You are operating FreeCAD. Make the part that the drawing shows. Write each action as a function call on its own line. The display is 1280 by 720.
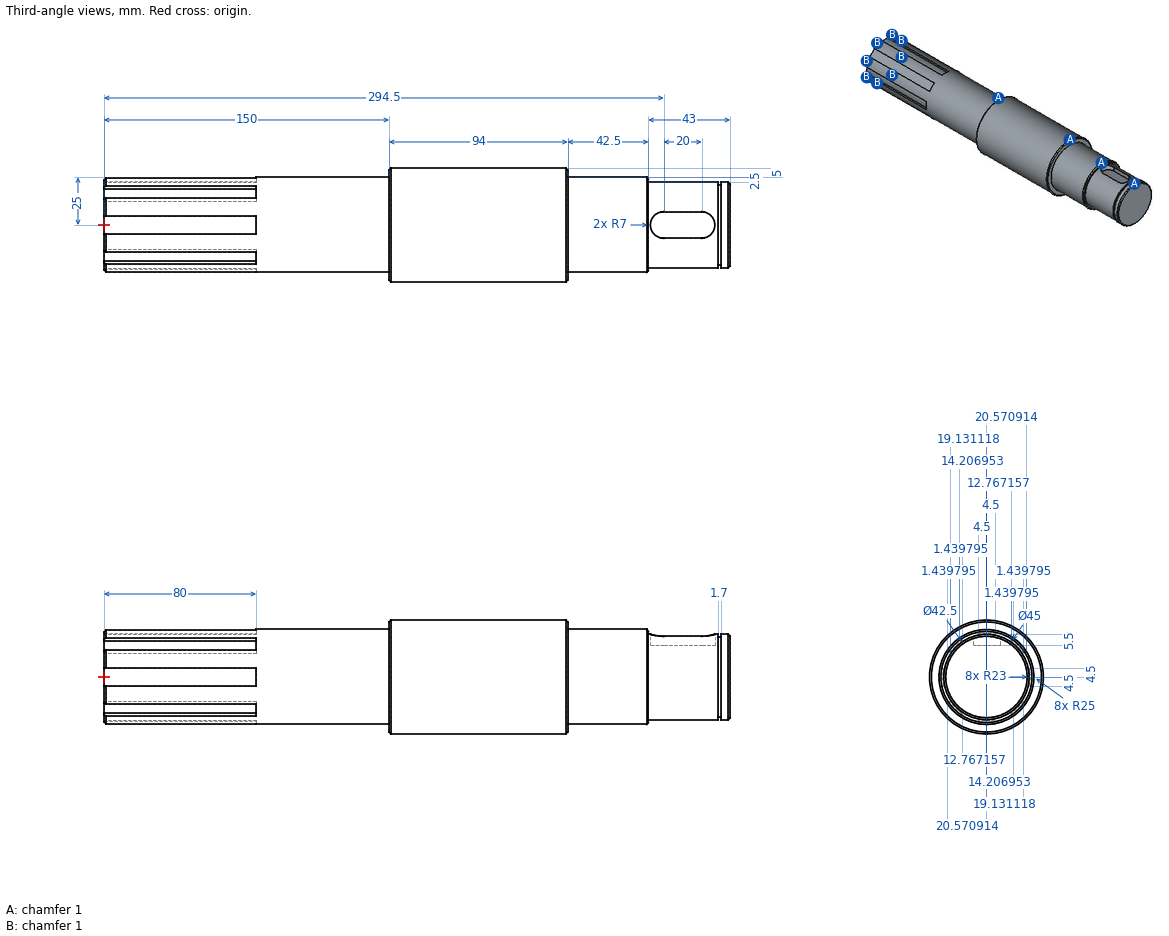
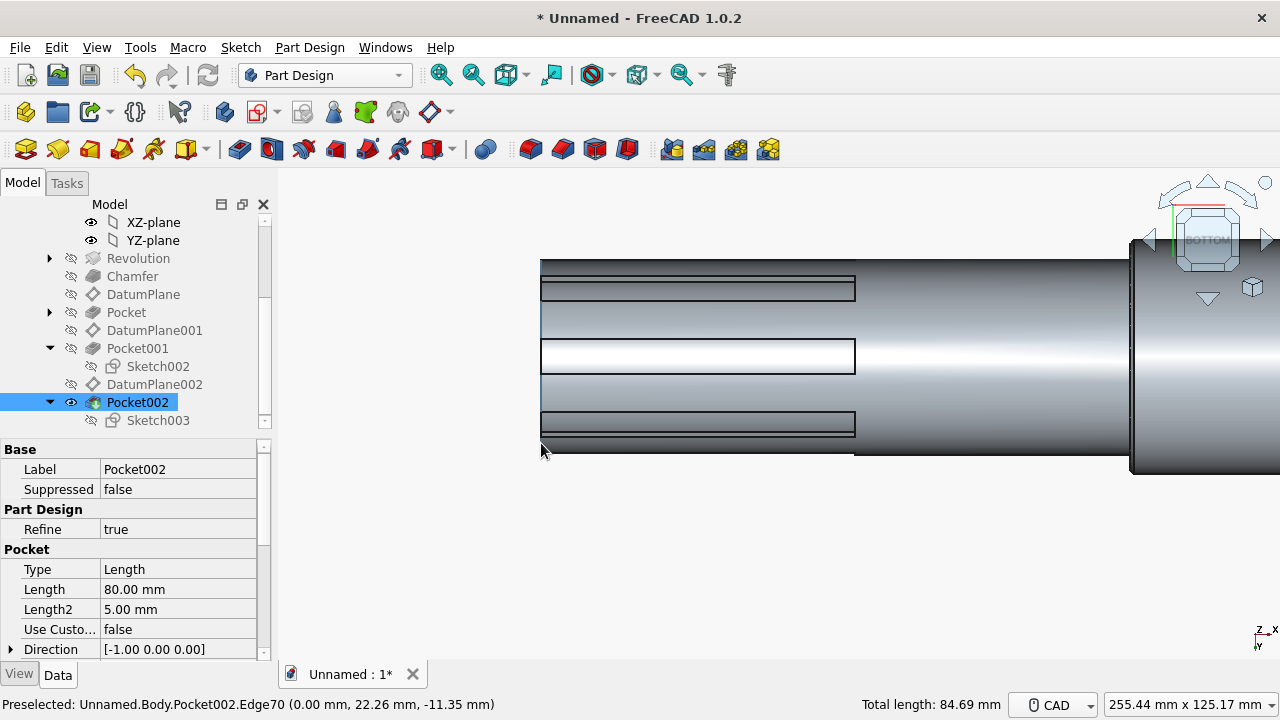
click(564, 150)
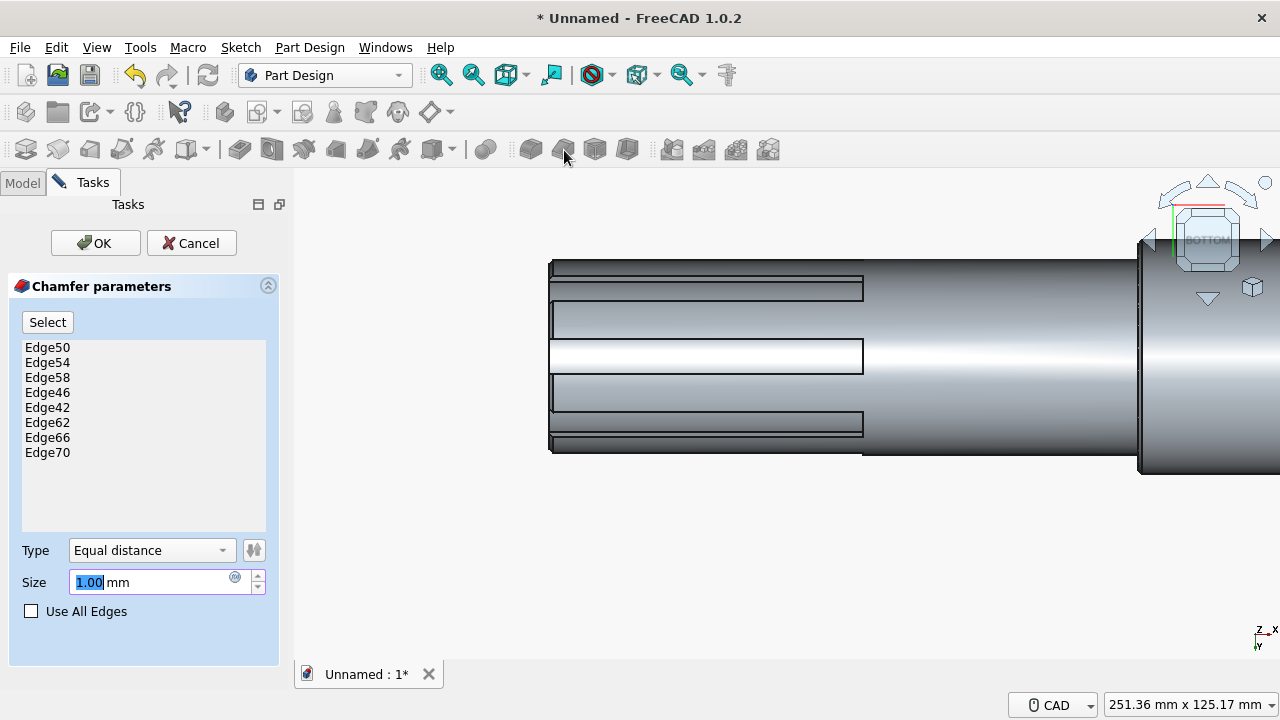
text(1)
key(Tab)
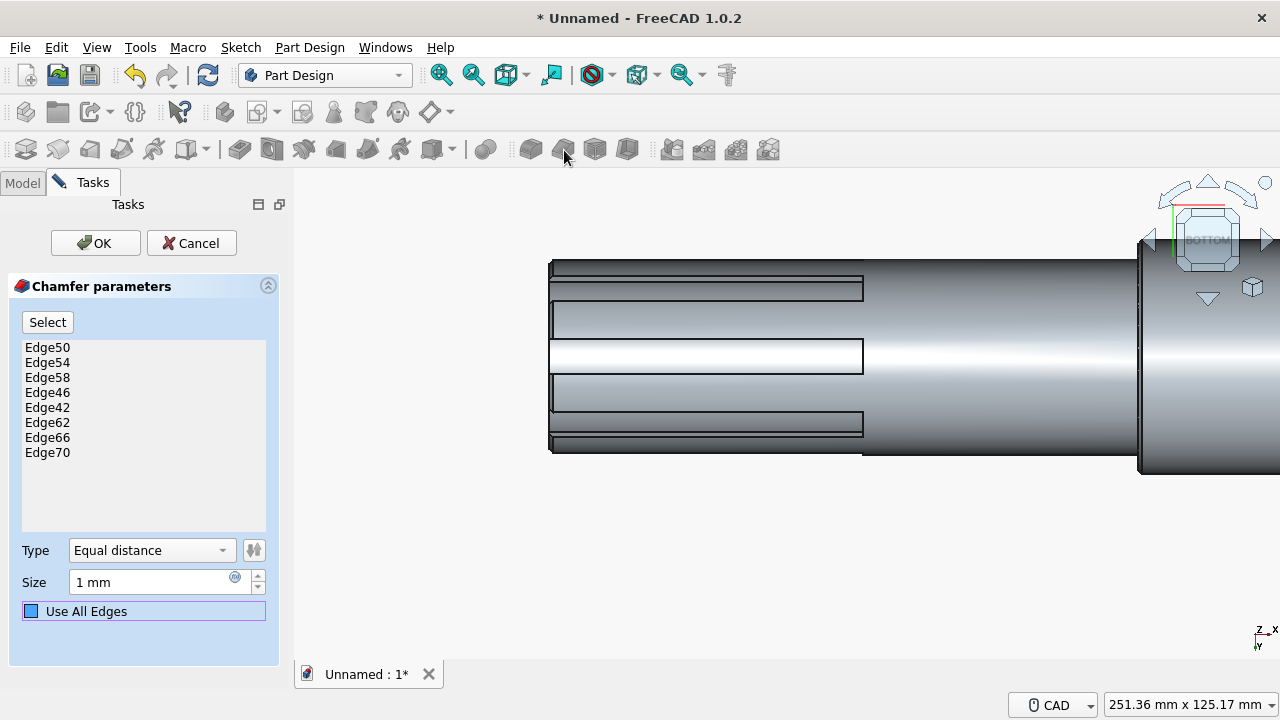
click(96, 243)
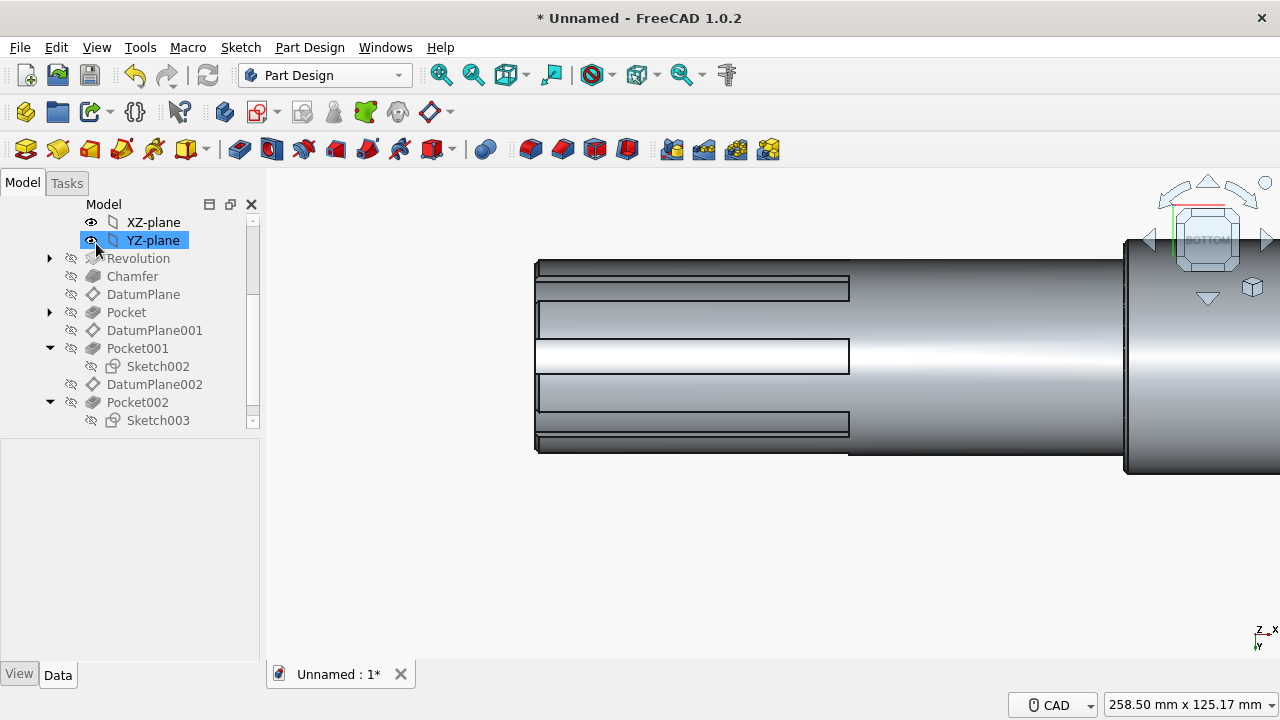
key(0)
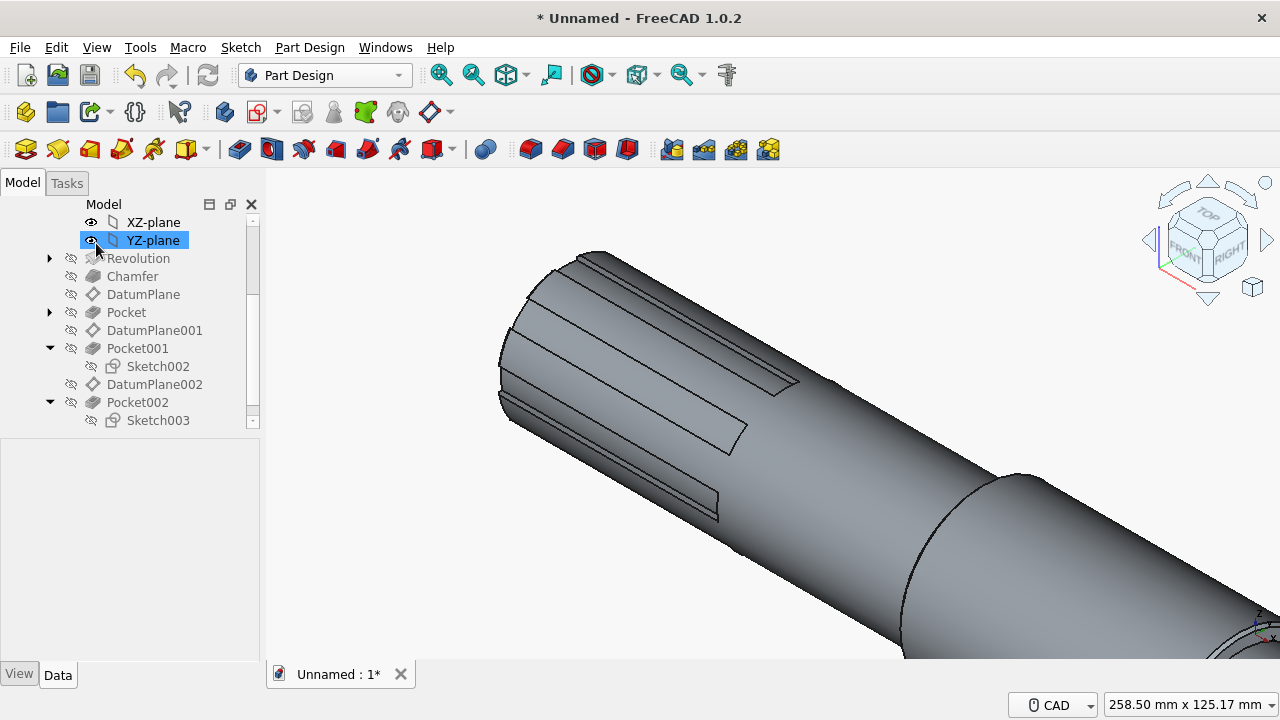
click(442, 76)